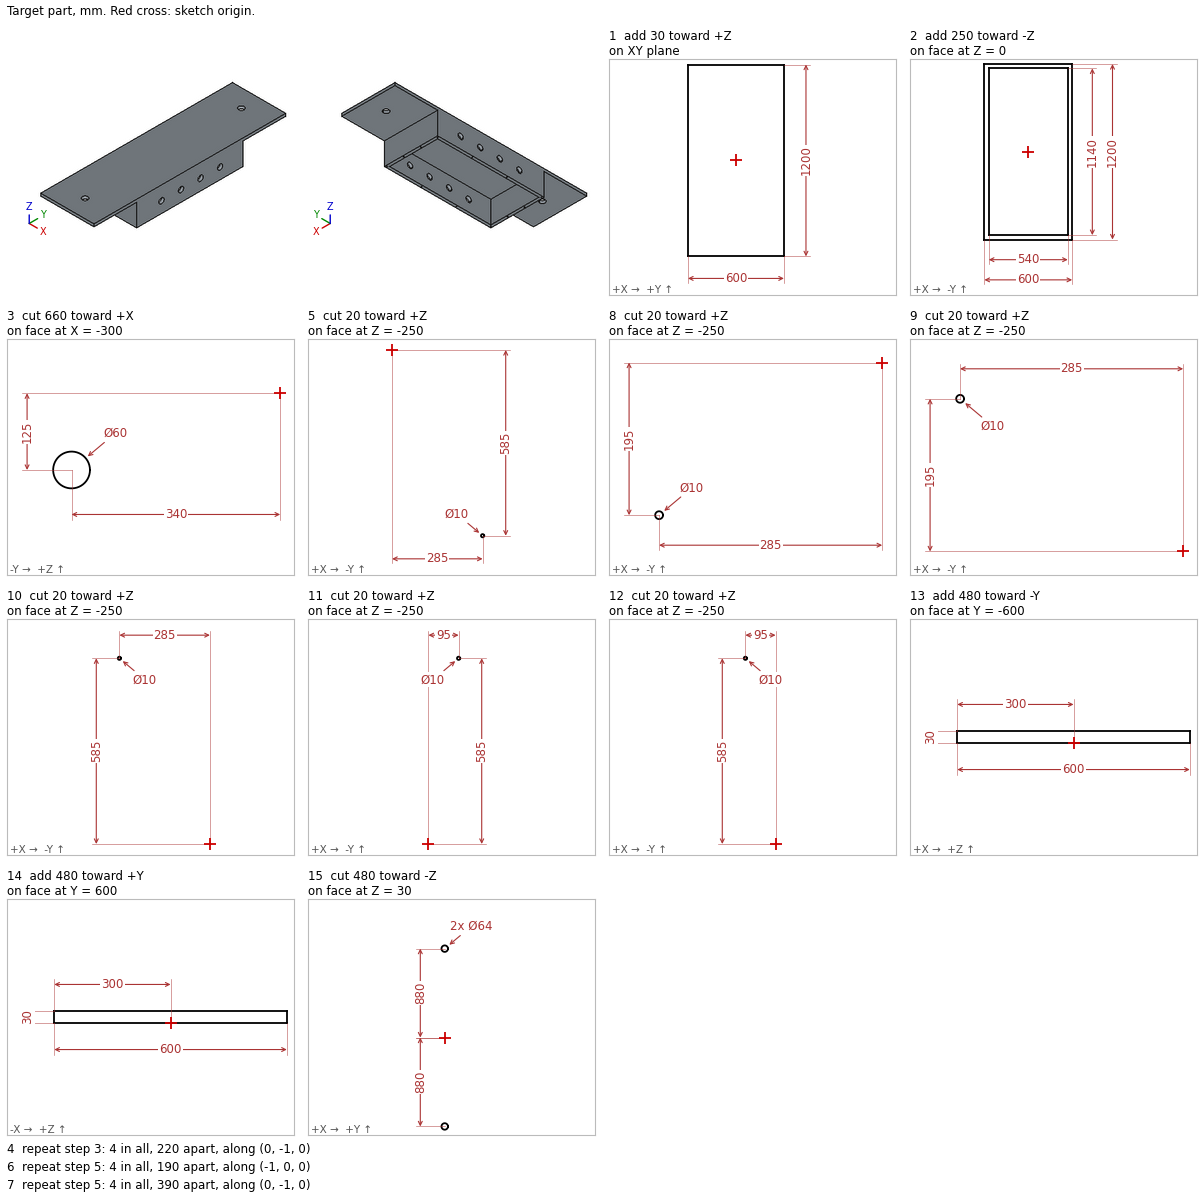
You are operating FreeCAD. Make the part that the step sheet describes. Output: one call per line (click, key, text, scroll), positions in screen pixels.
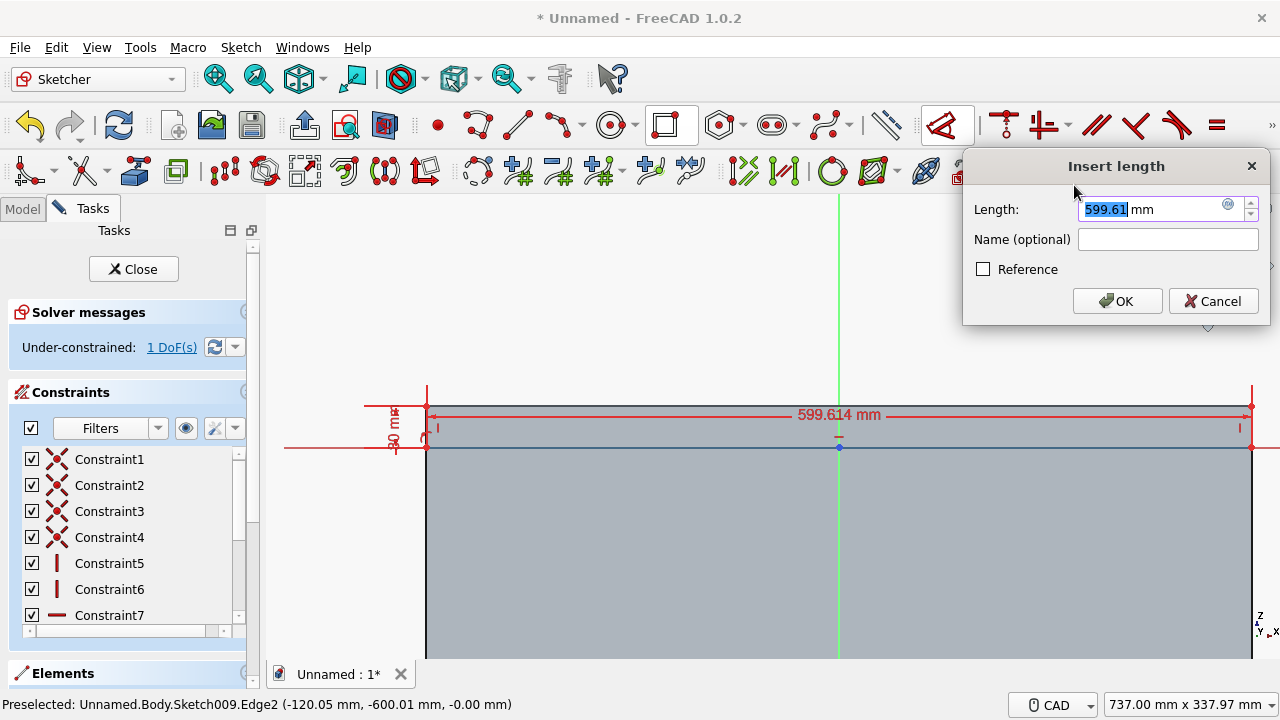
text(600)
key(Return)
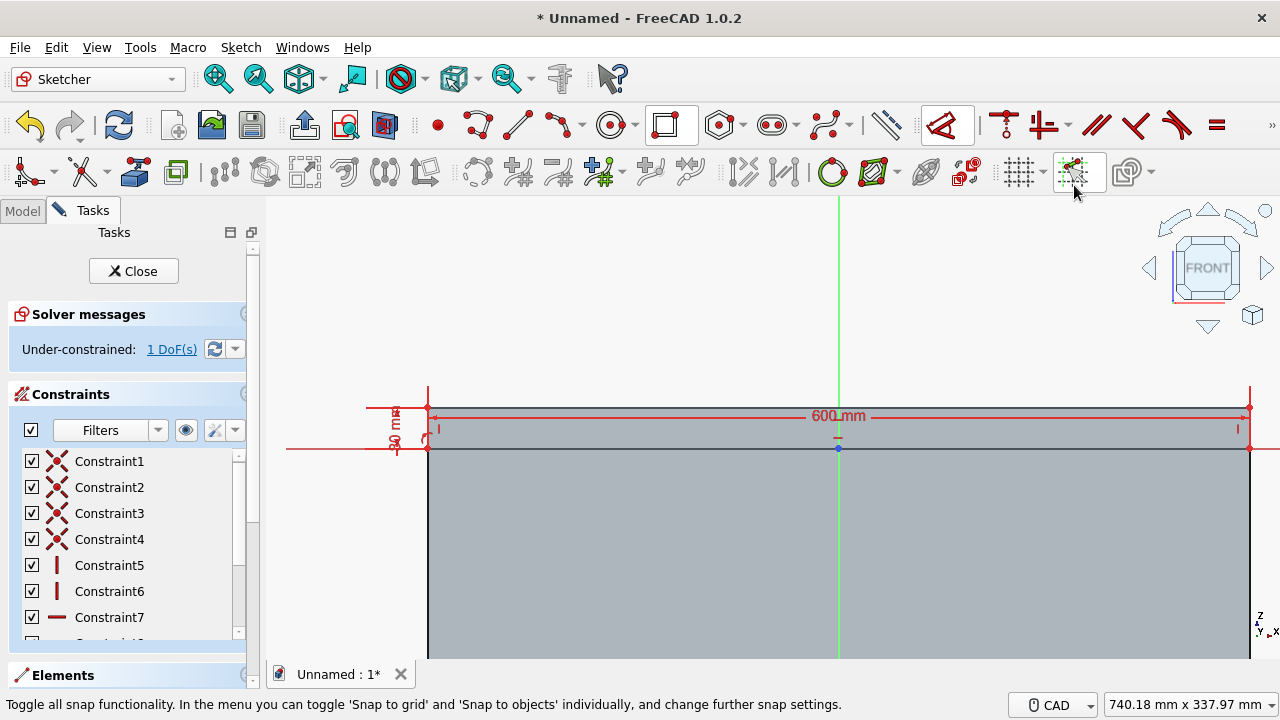
click(428, 408)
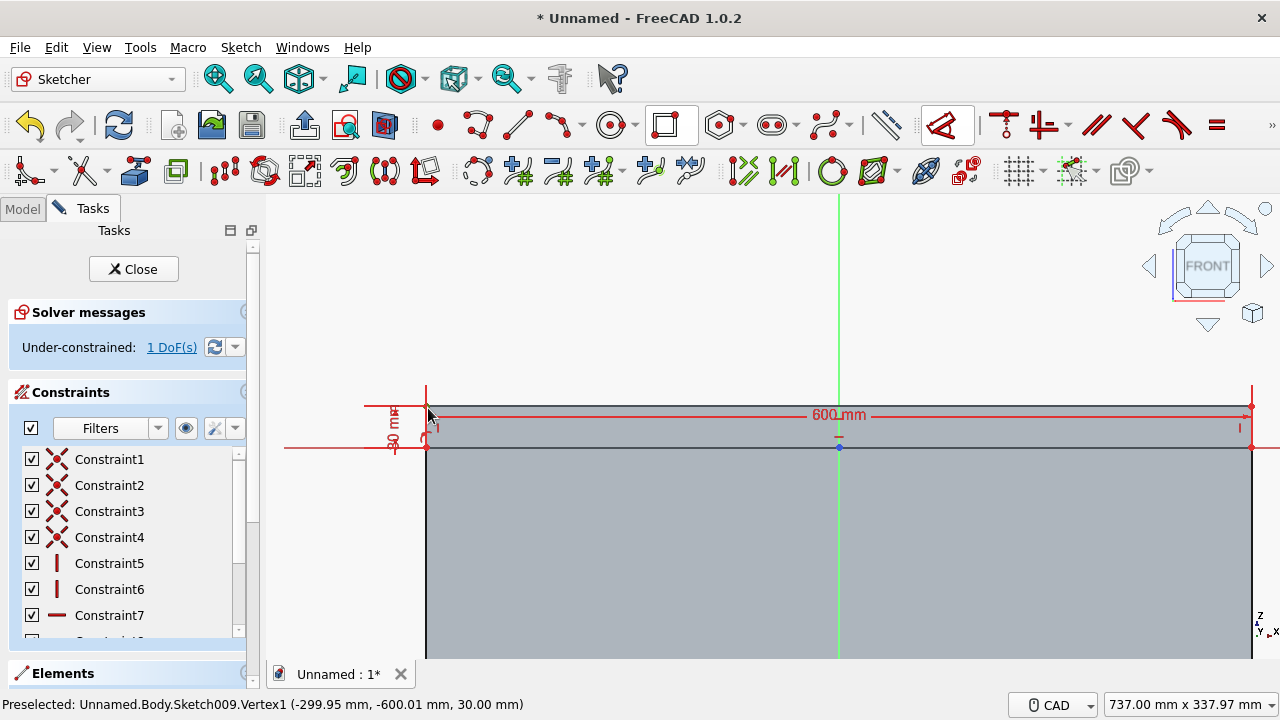
click(968, 126)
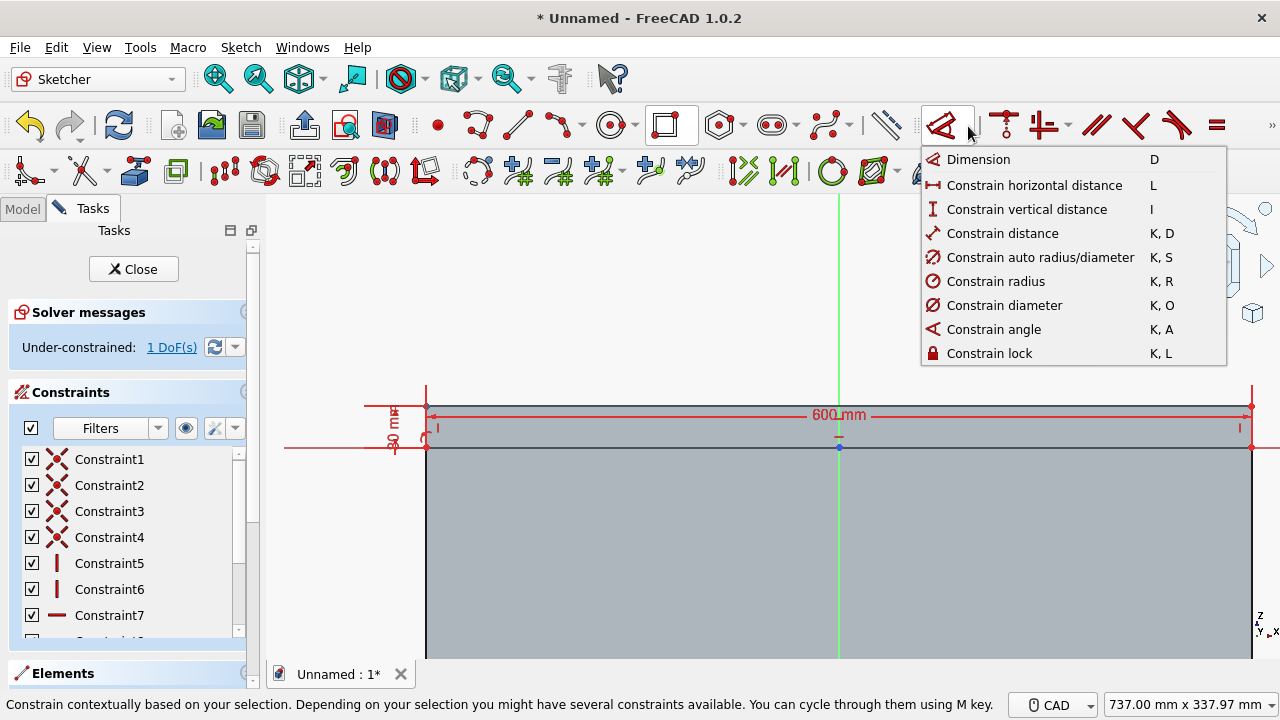
click(1074, 185)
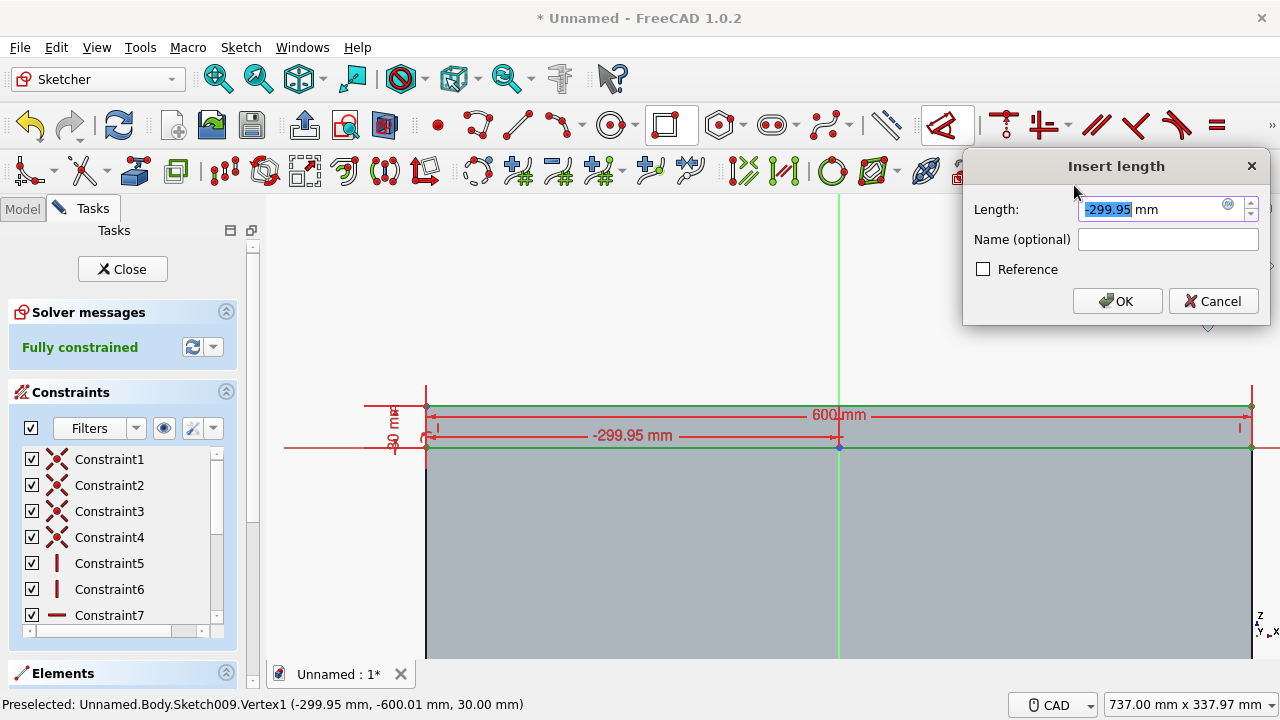
text(-300)
key(Return)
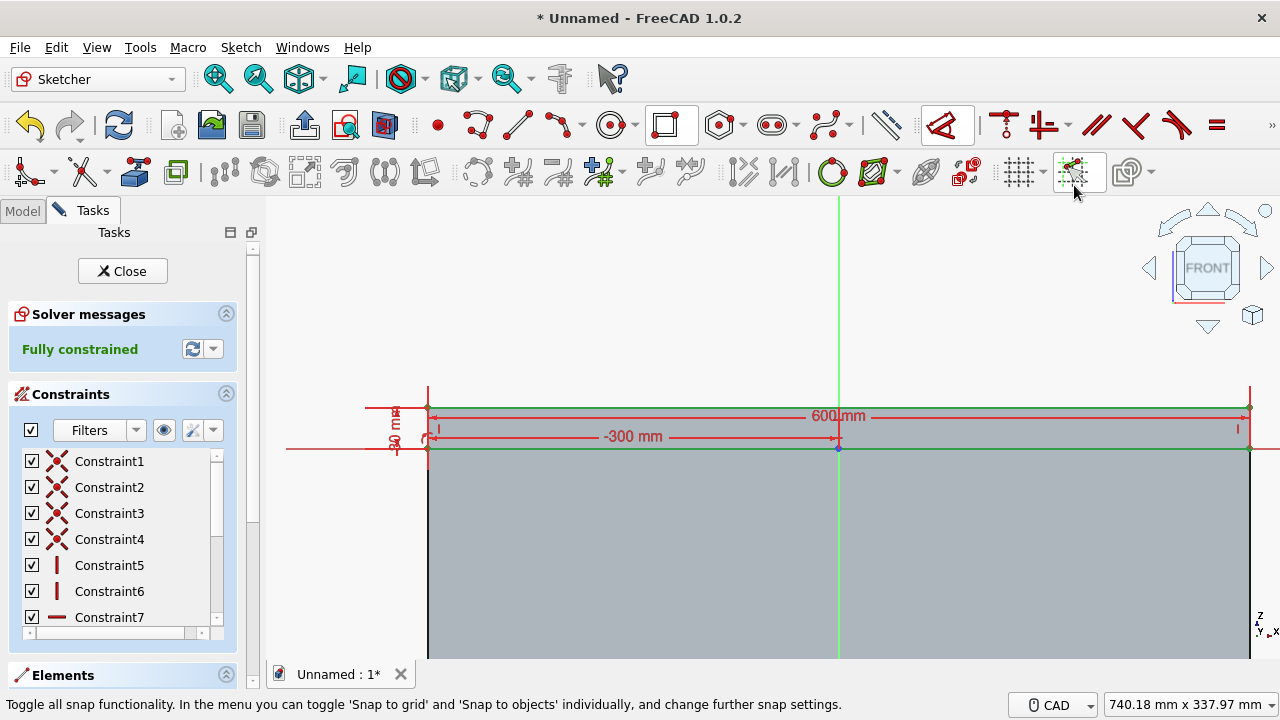
click(123, 271)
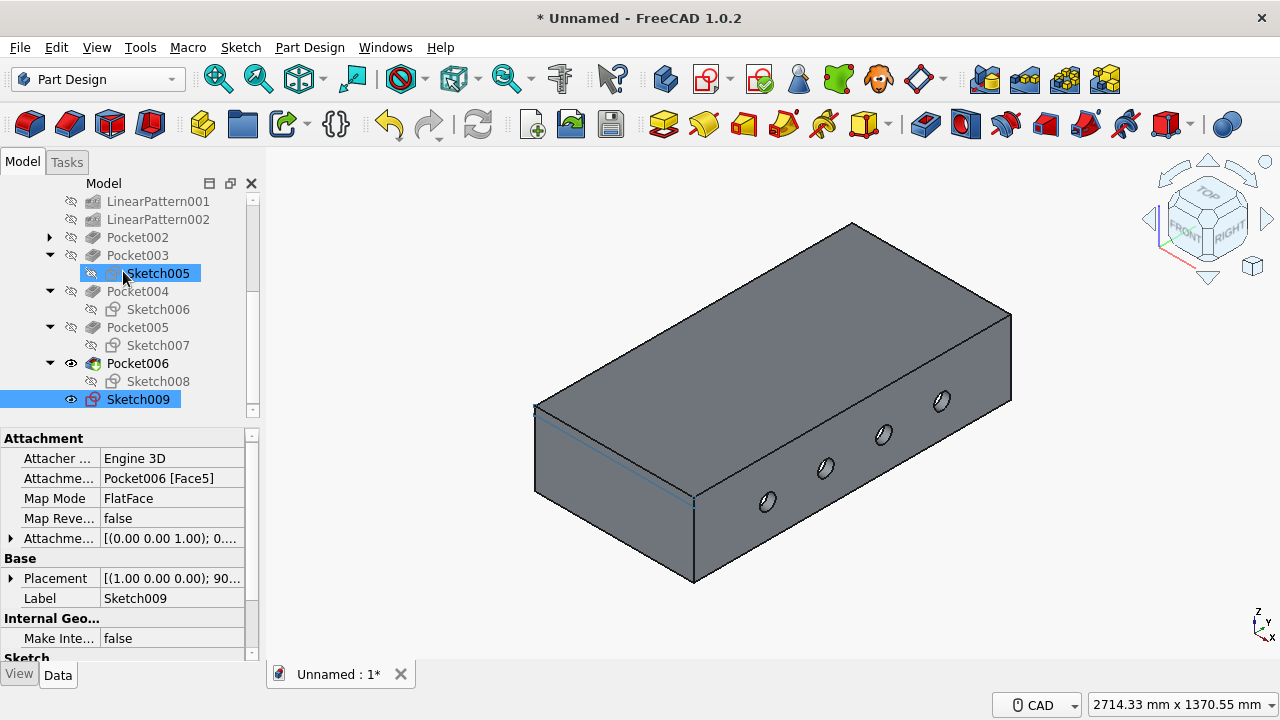
click(664, 124)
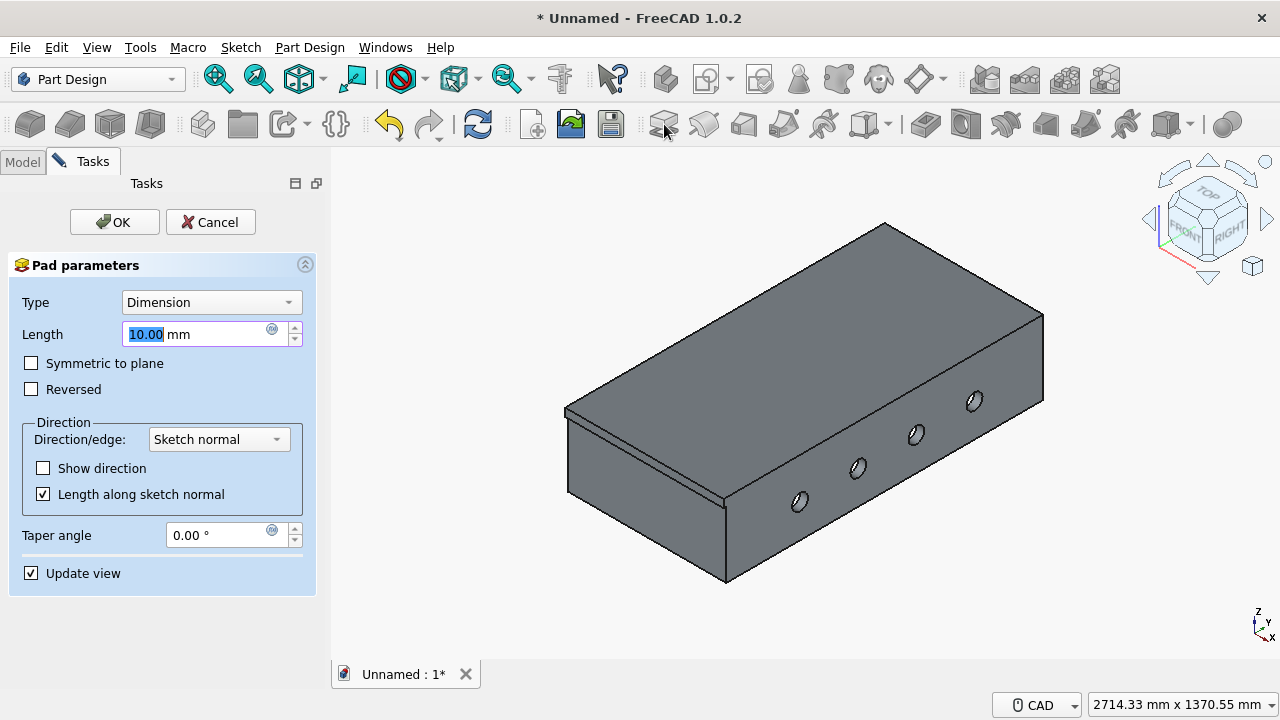
text(480)
key(Tab)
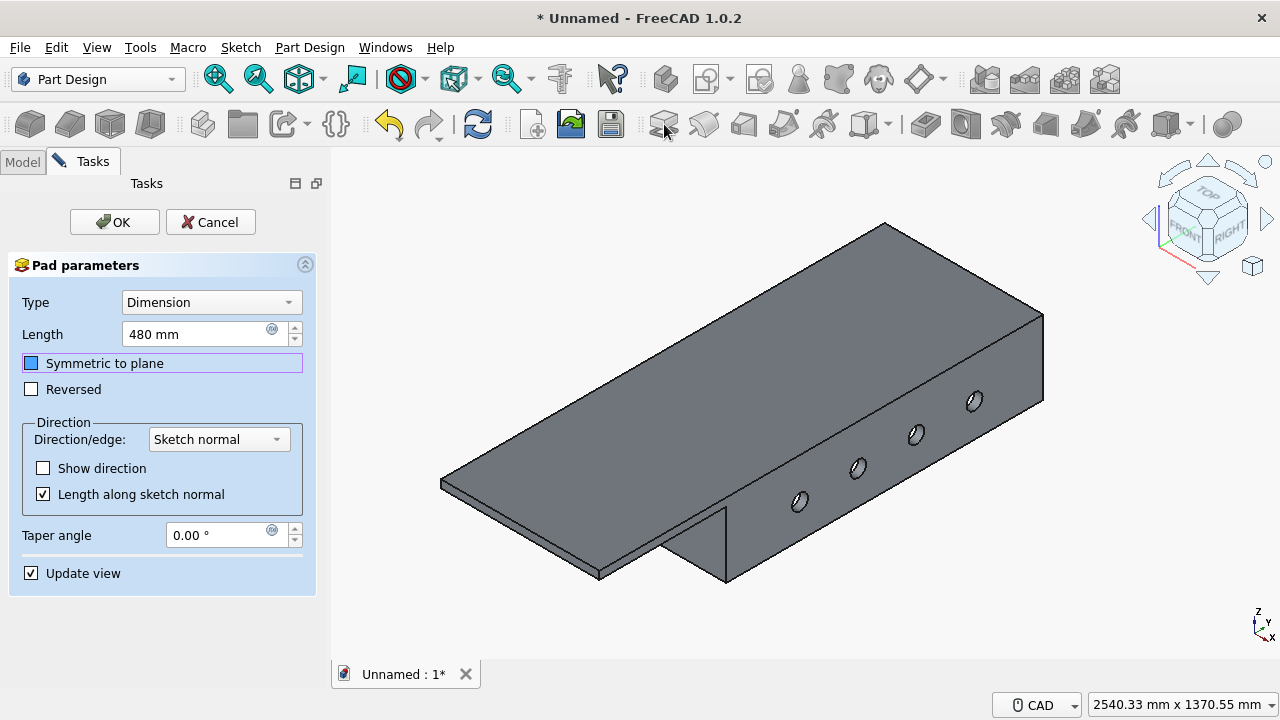
click(115, 222)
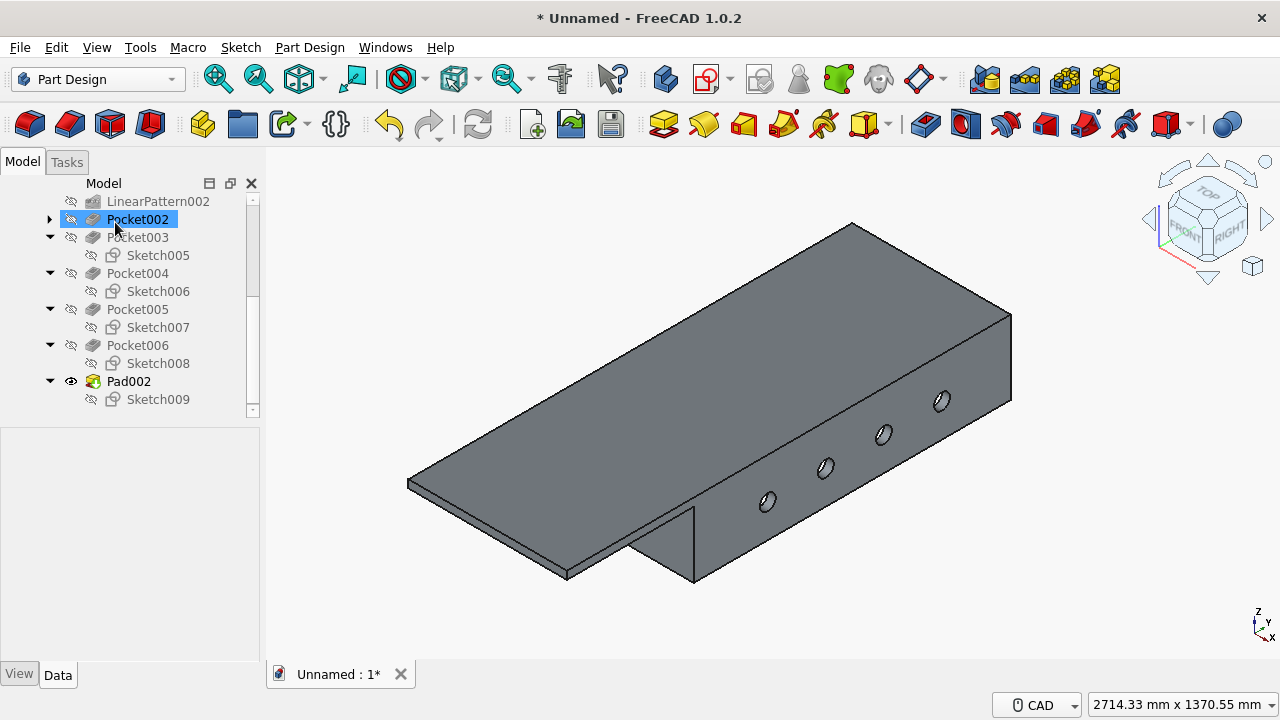
key(4)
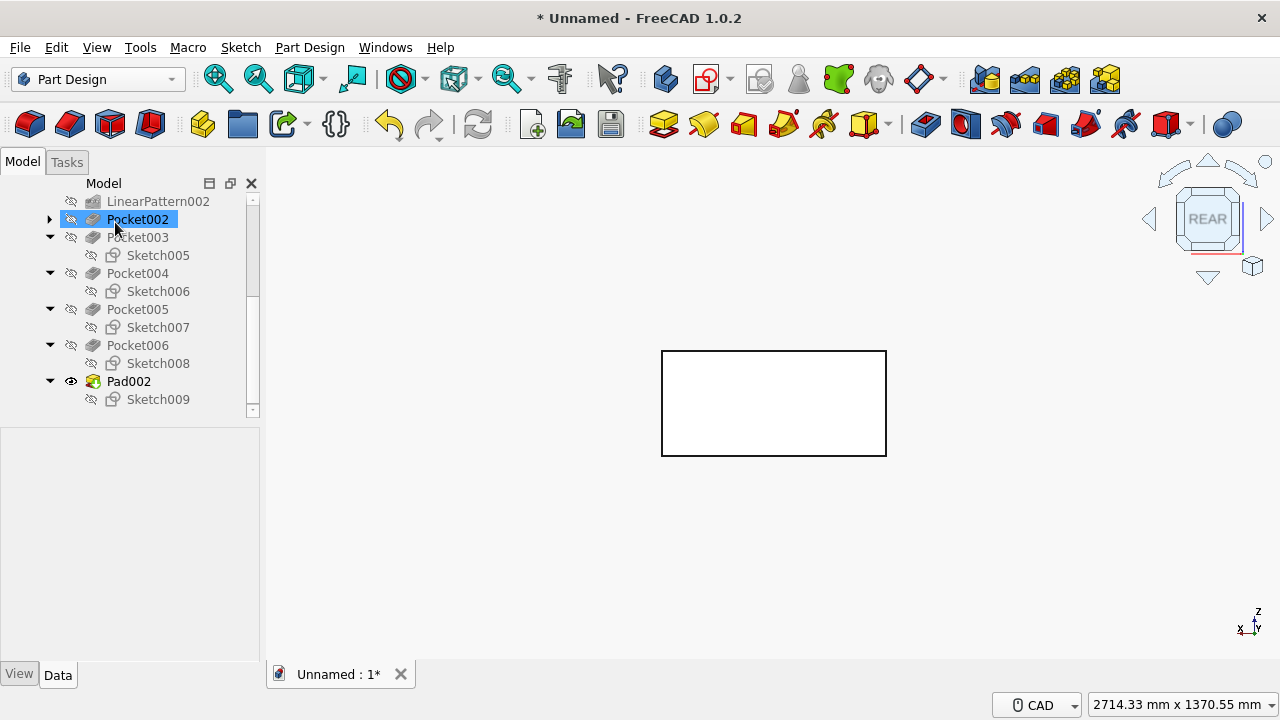
click(220, 80)